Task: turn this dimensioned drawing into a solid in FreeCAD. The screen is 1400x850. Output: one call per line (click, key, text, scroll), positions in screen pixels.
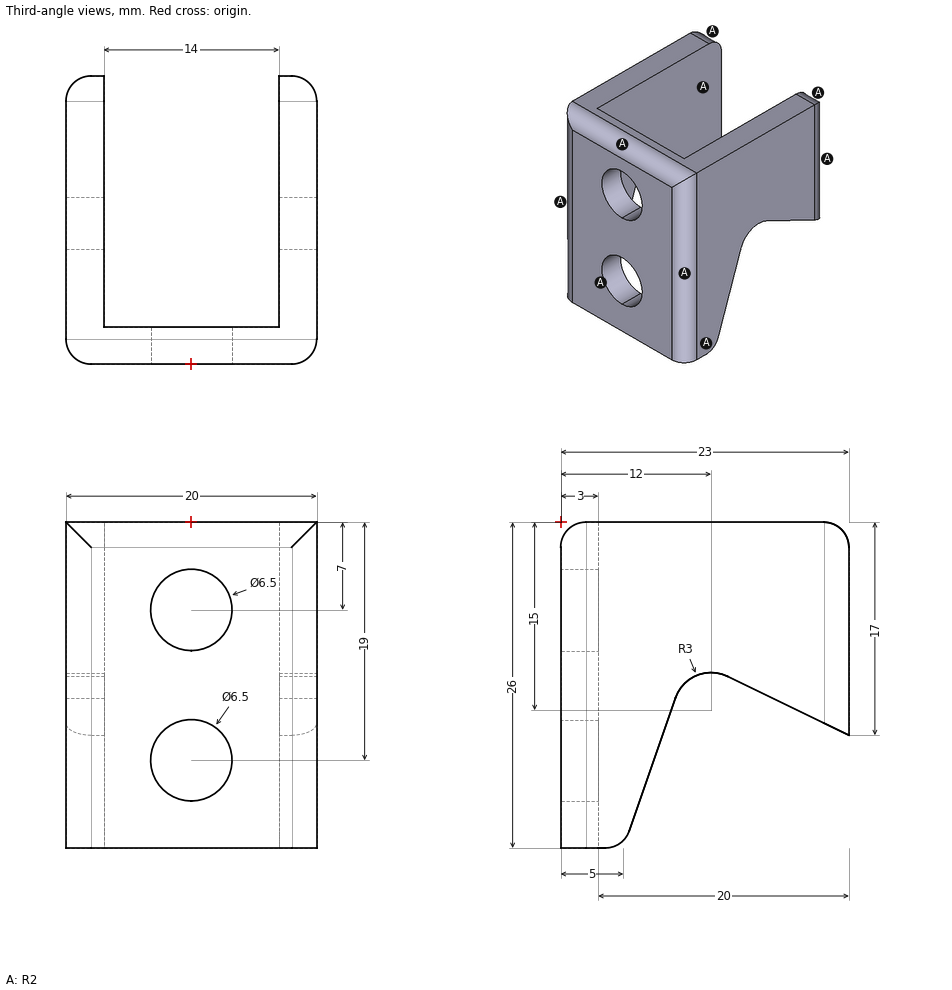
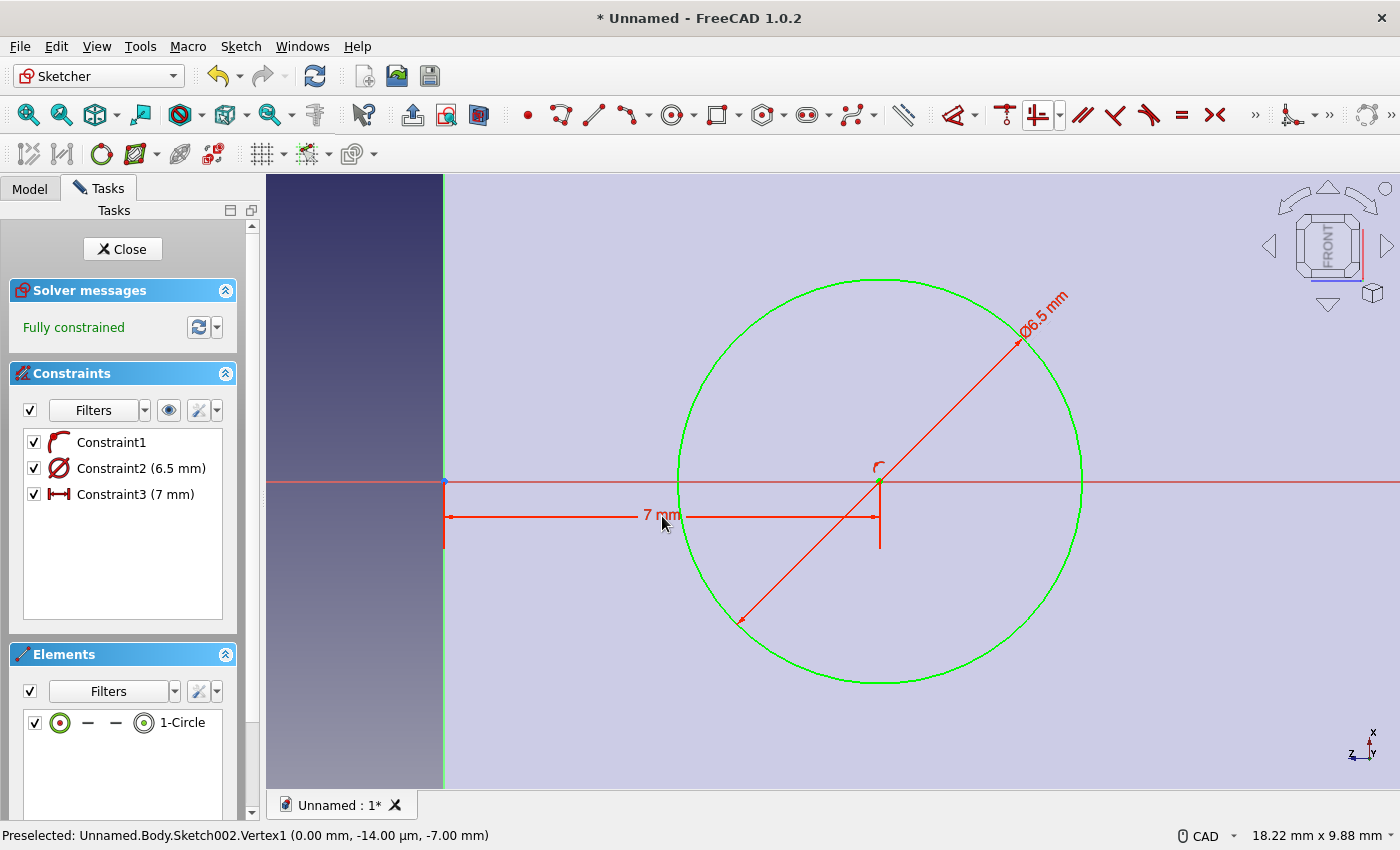
click(123, 249)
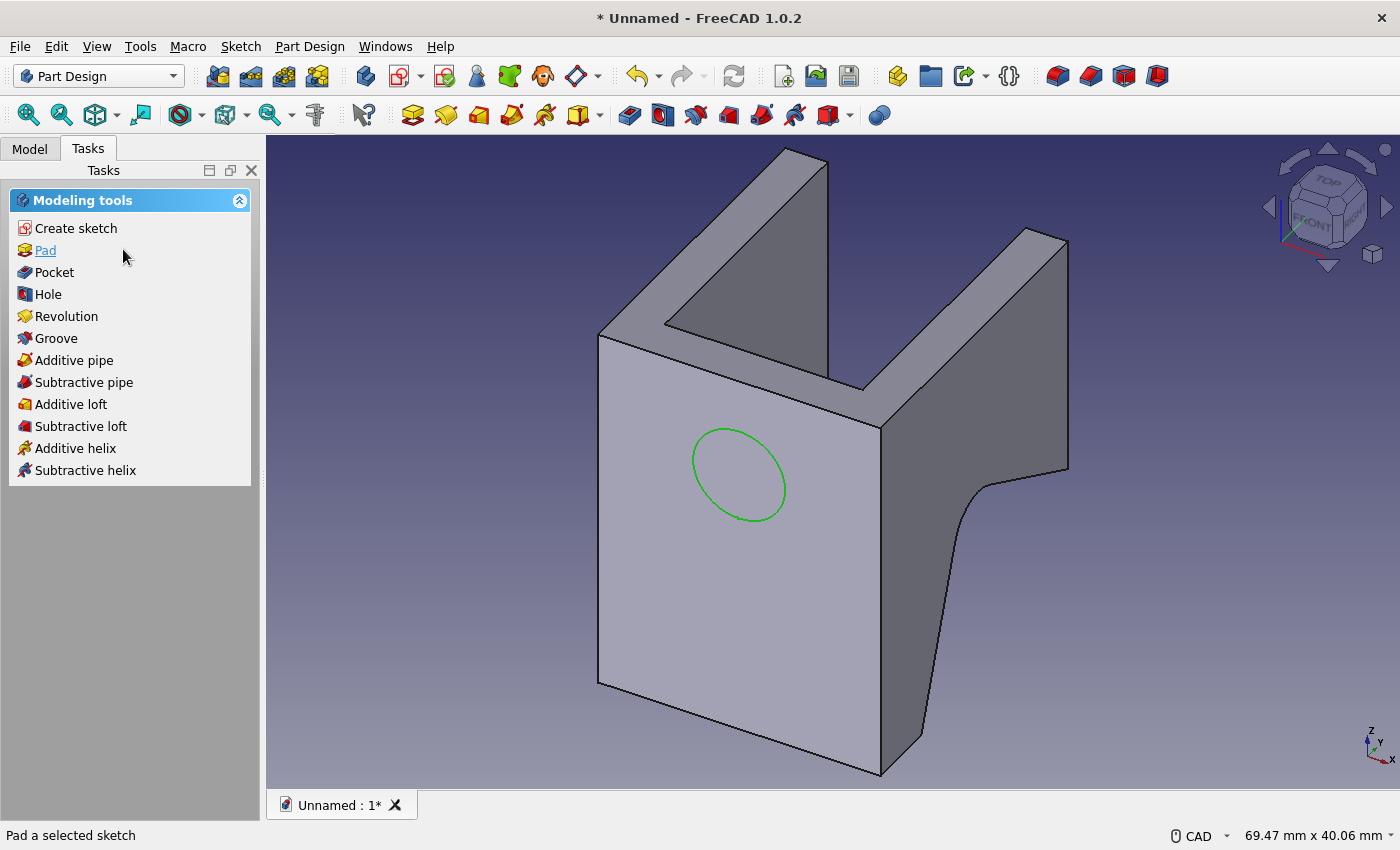
click(630, 116)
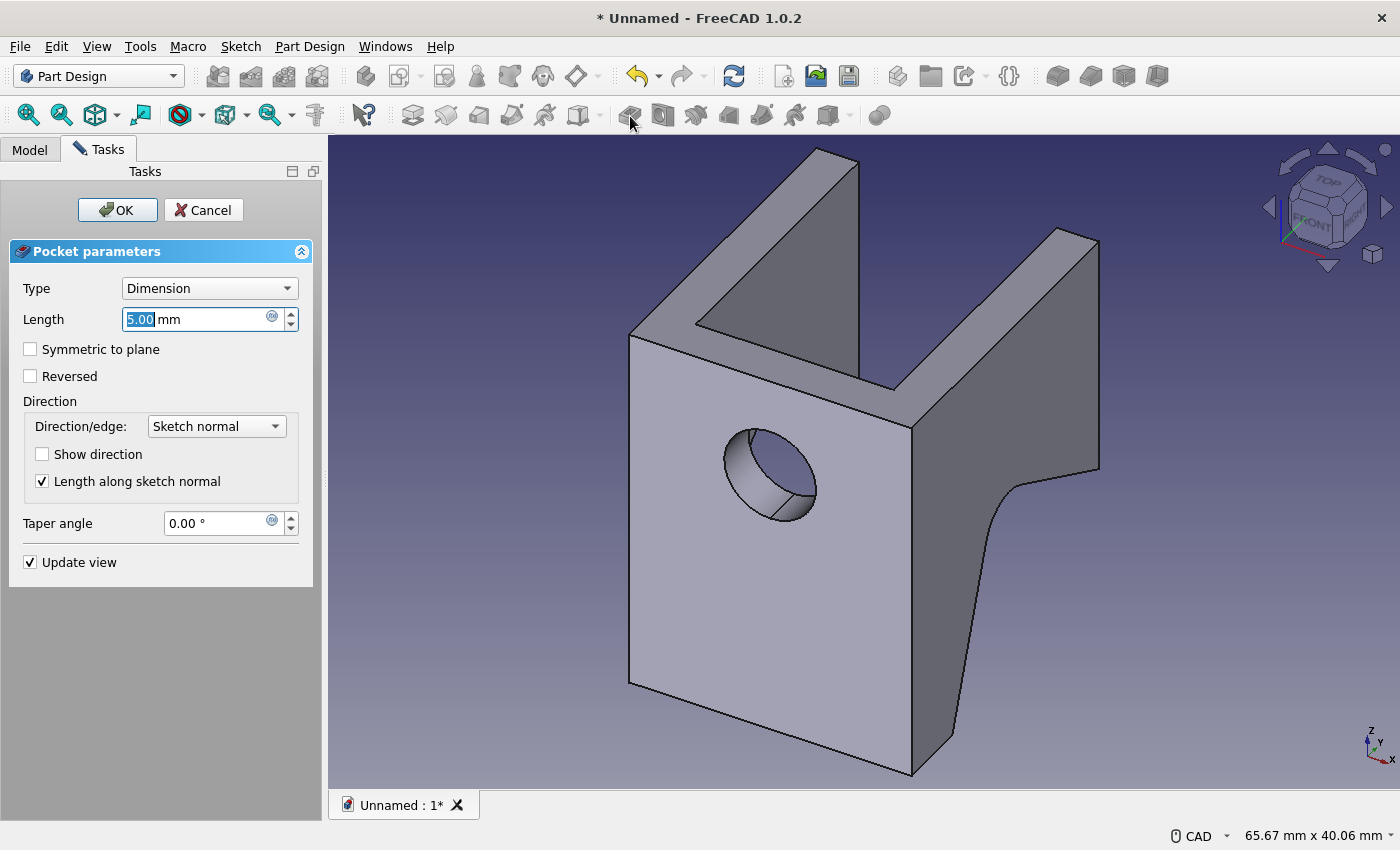
click(210, 288)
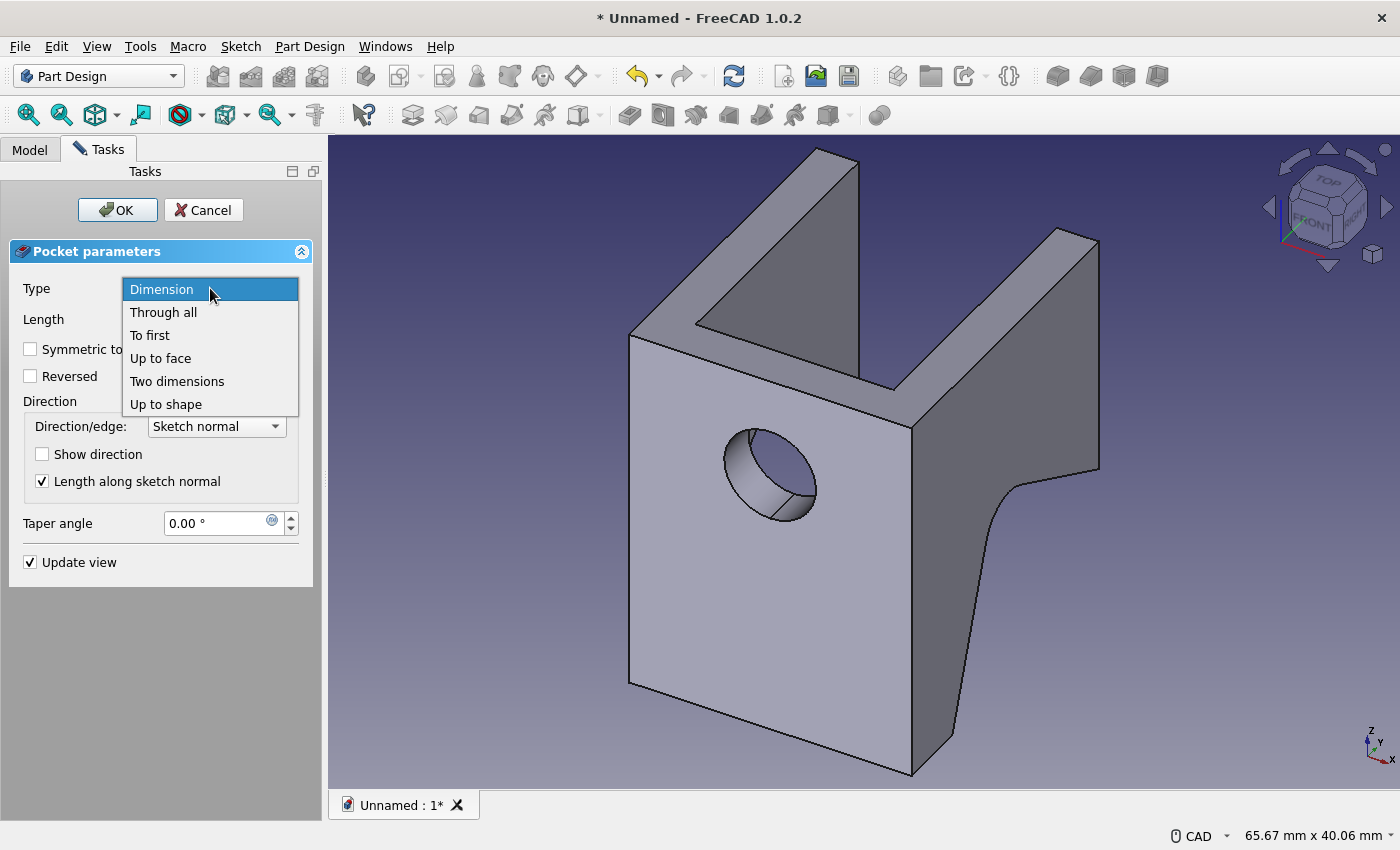
click(208, 336)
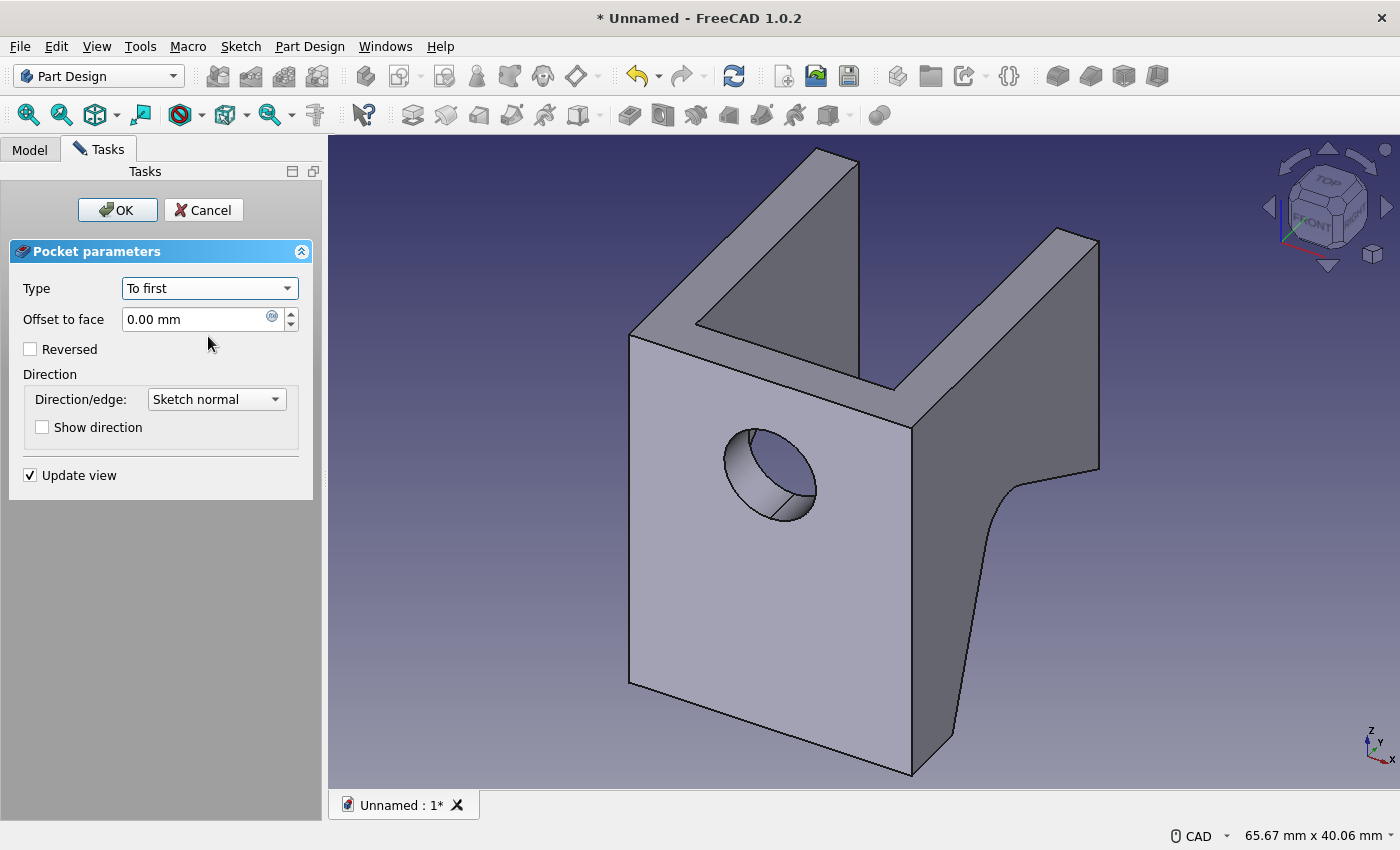
click(118, 210)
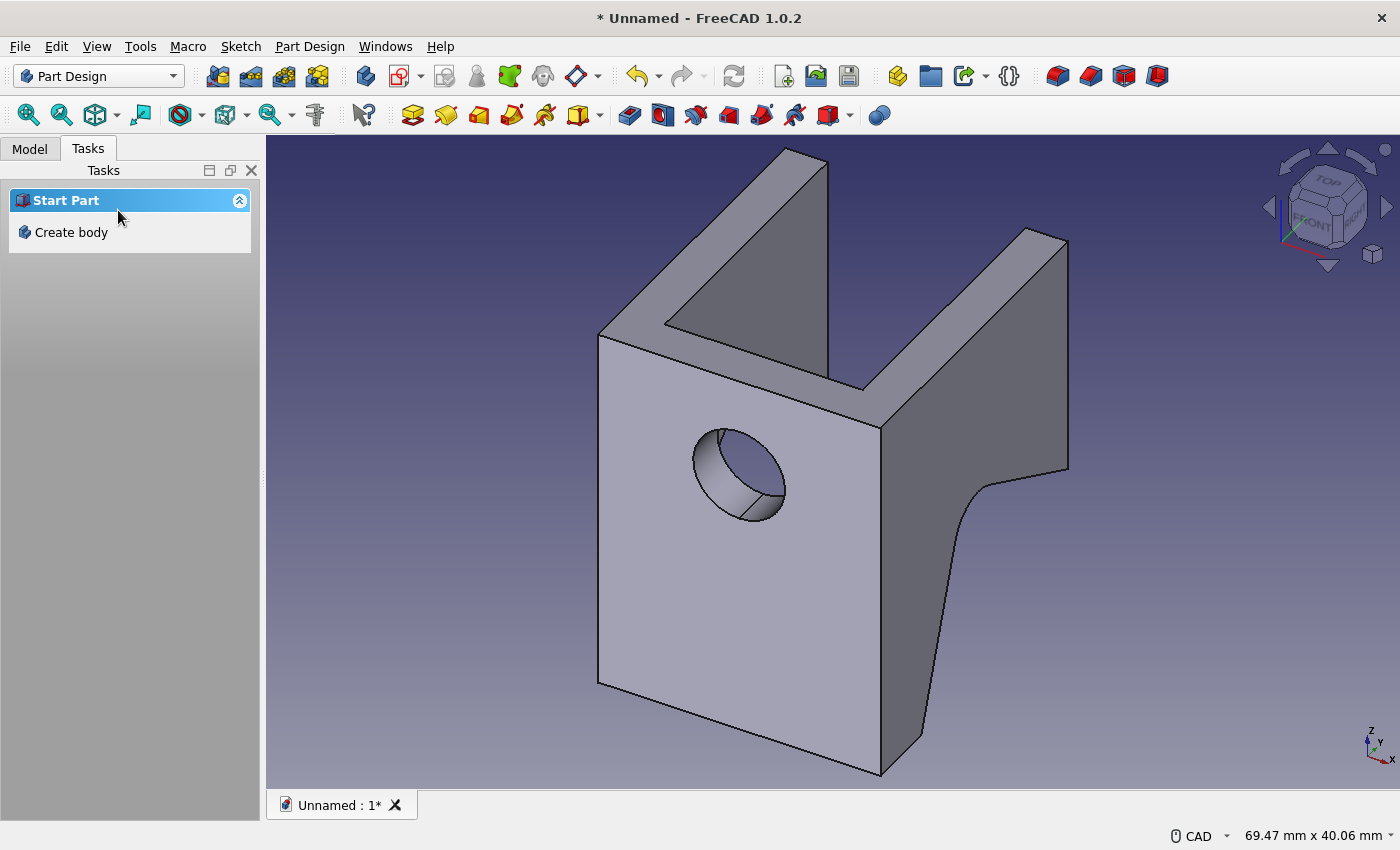
click(780, 617)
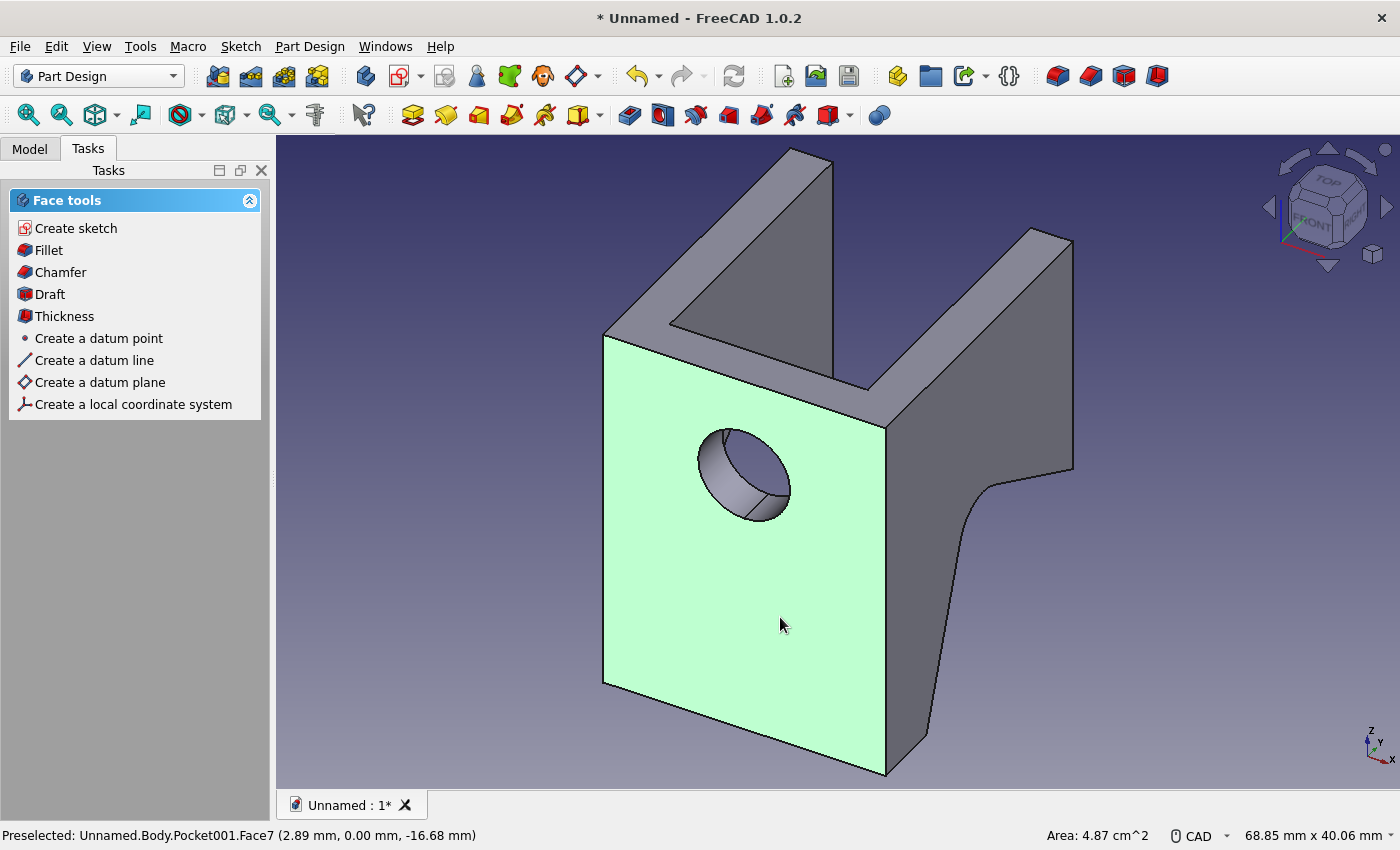
click(398, 76)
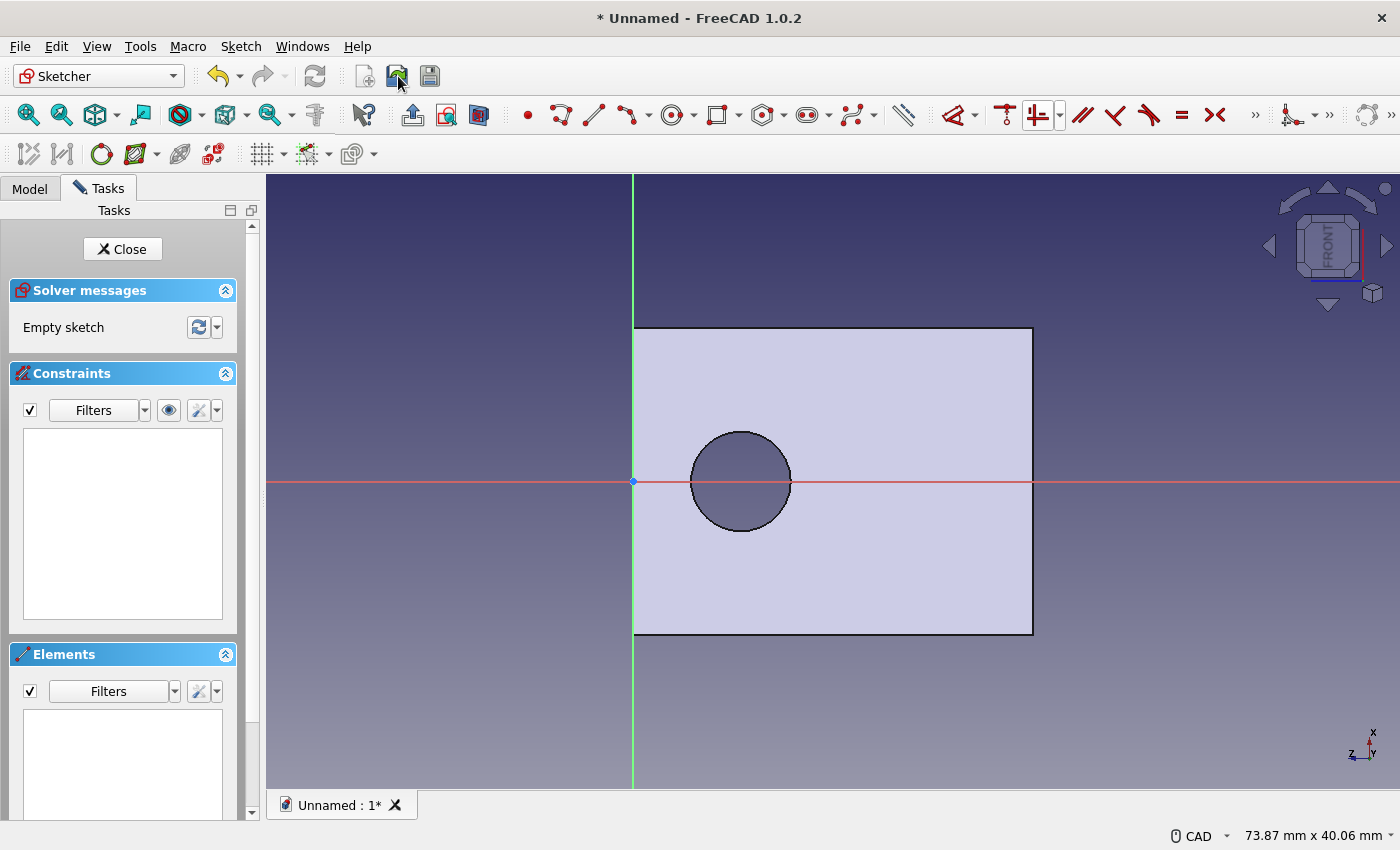
scroll(978, 481, up, 7)